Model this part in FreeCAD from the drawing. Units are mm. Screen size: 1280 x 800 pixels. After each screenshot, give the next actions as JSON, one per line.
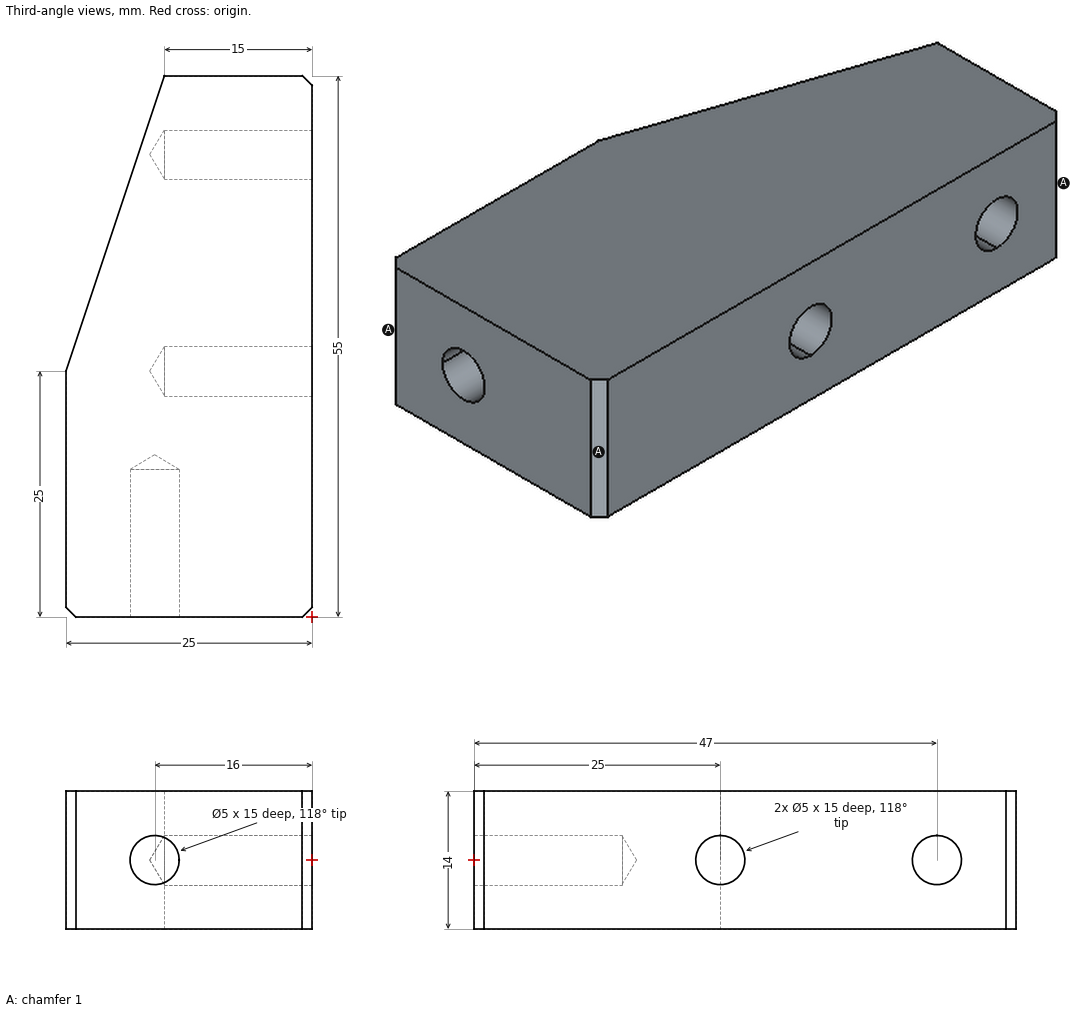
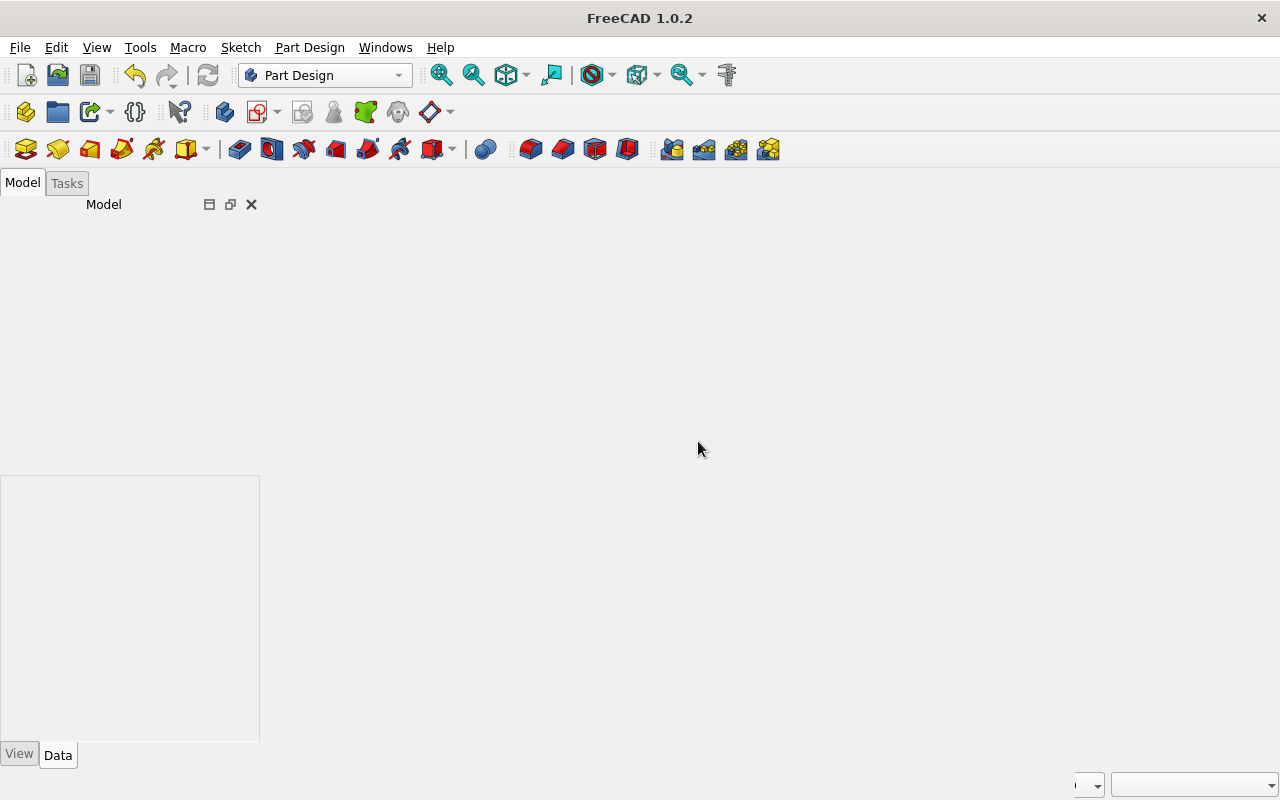
{"action": "key", "text": "ctrl+n"}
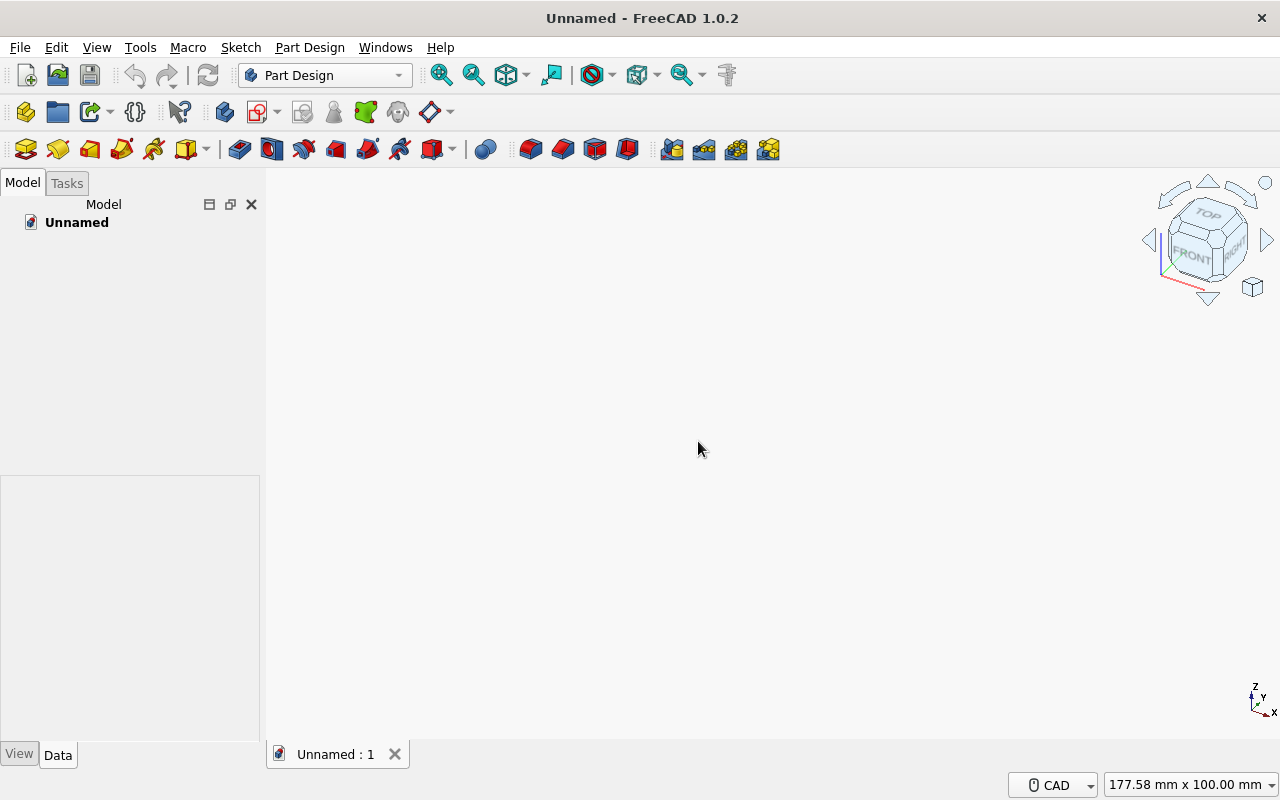
{"action": "left_click", "coordinate": [258, 112]}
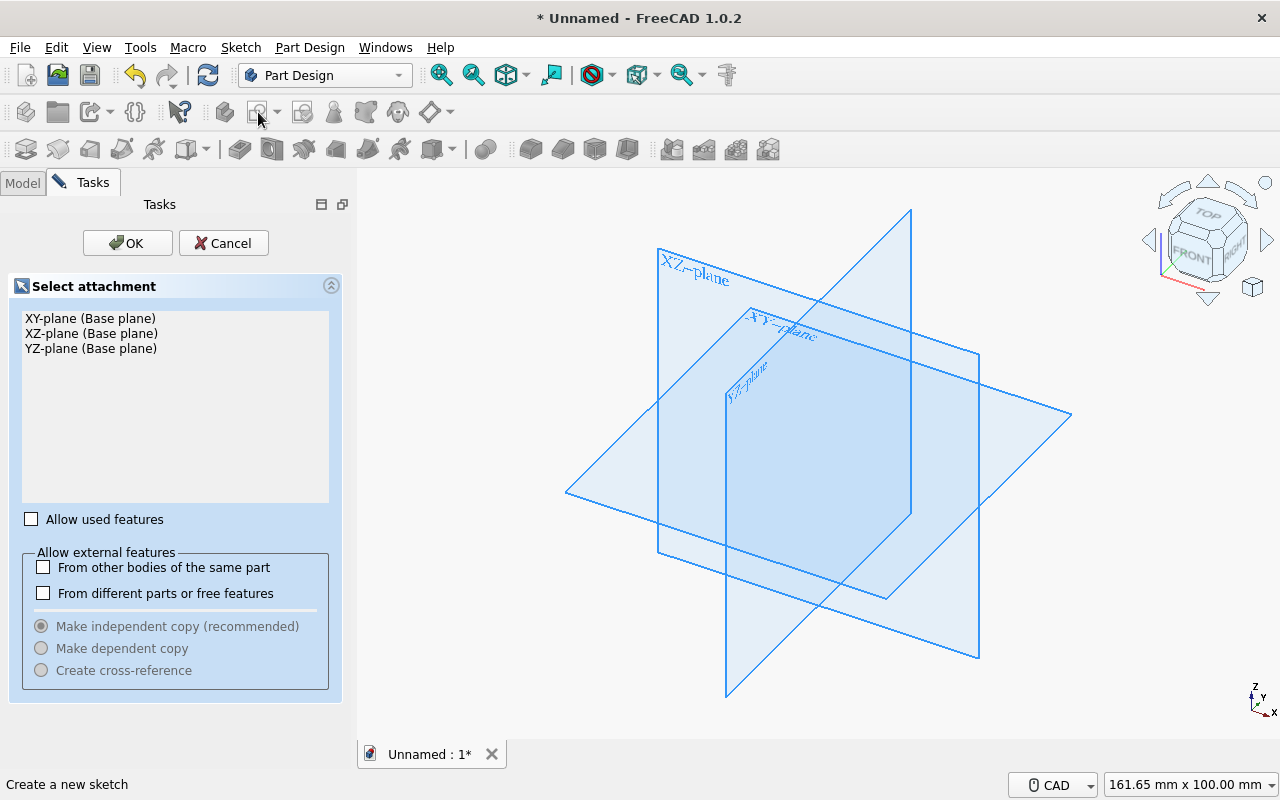
{"action": "left_click", "coordinate": [82, 318]}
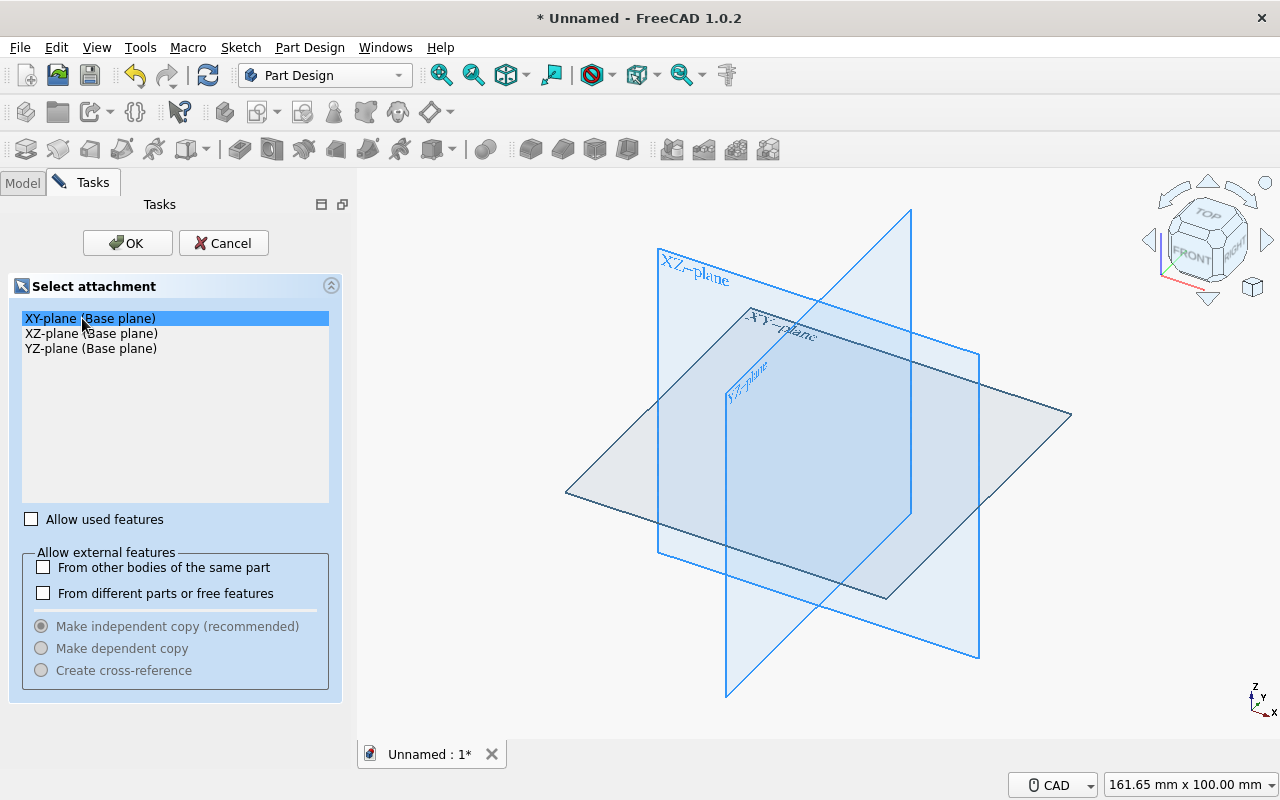
{"action": "left_click", "coordinate": [128, 243]}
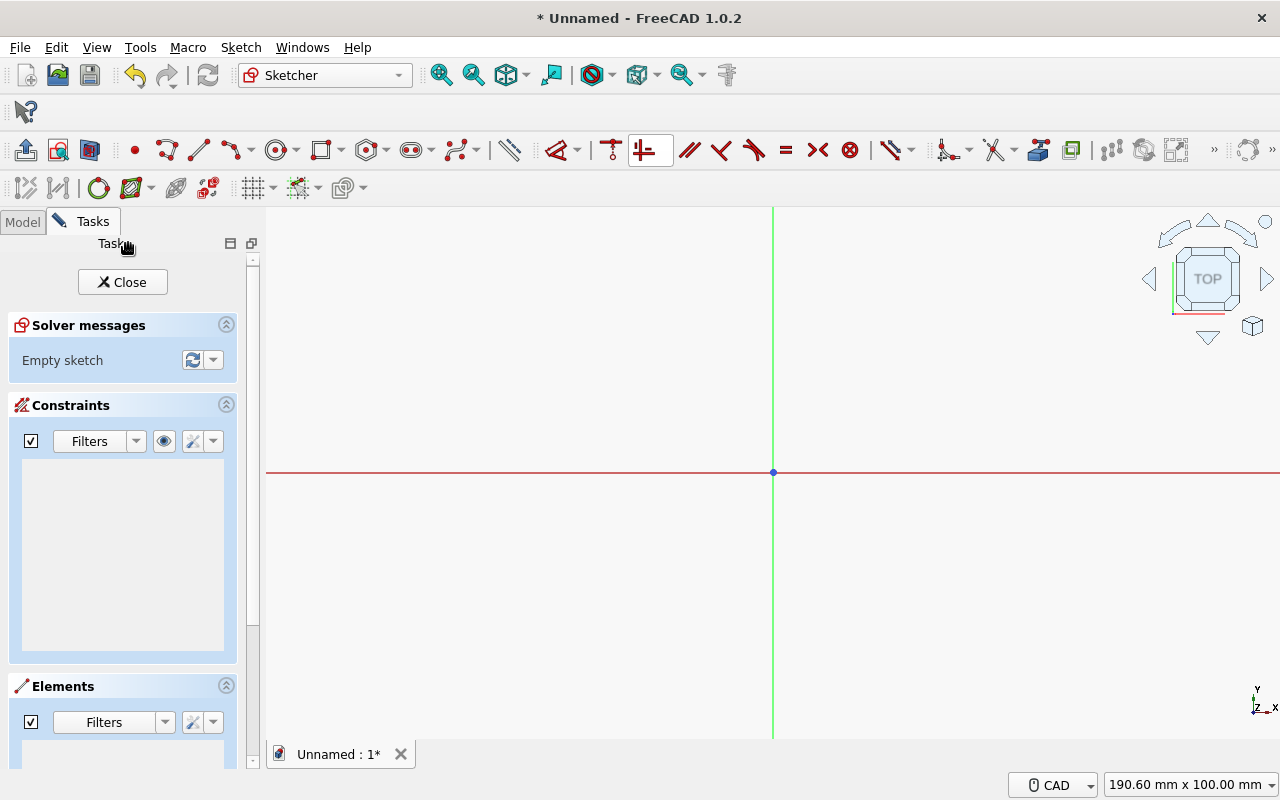
{"action": "scroll", "coordinate": [695, 711], "scroll_direction": "down", "scroll_amount": 1}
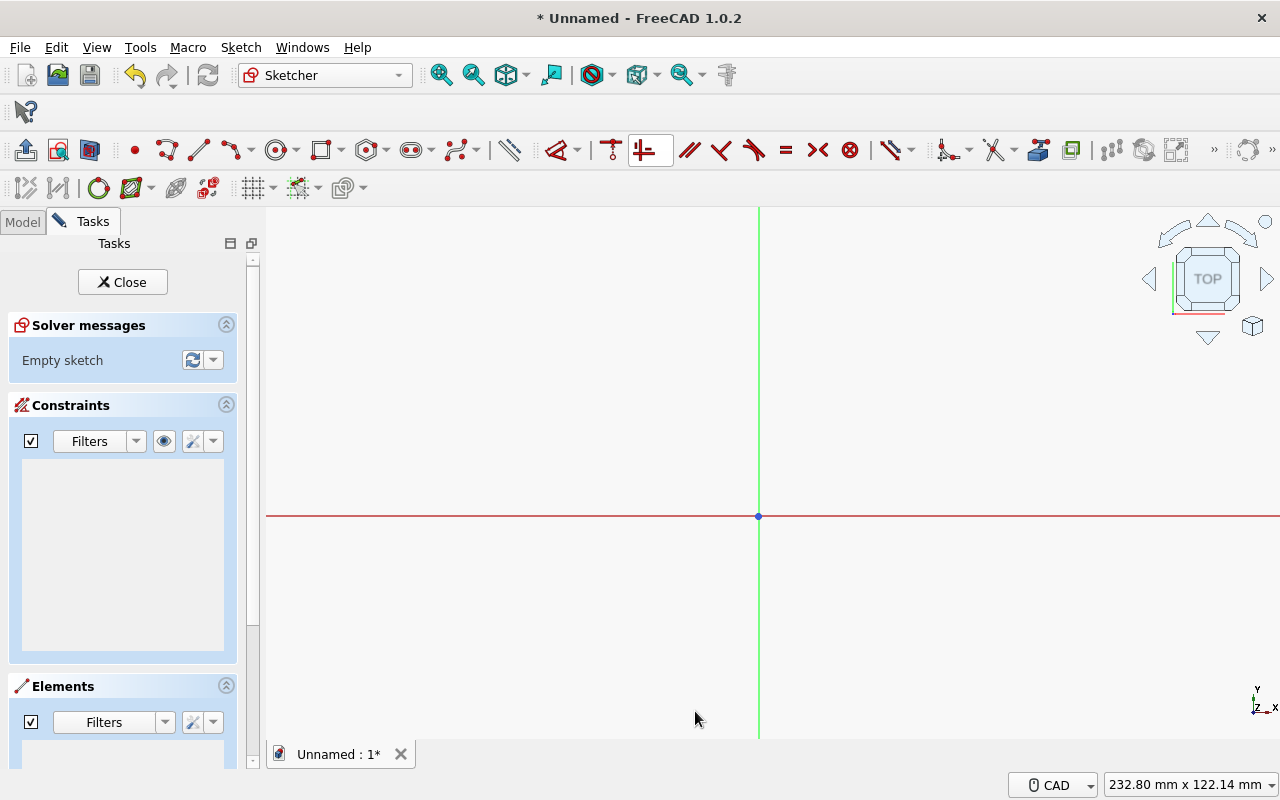
{"action": "scroll", "coordinate": [704, 241], "scroll_direction": "up", "scroll_amount": 2}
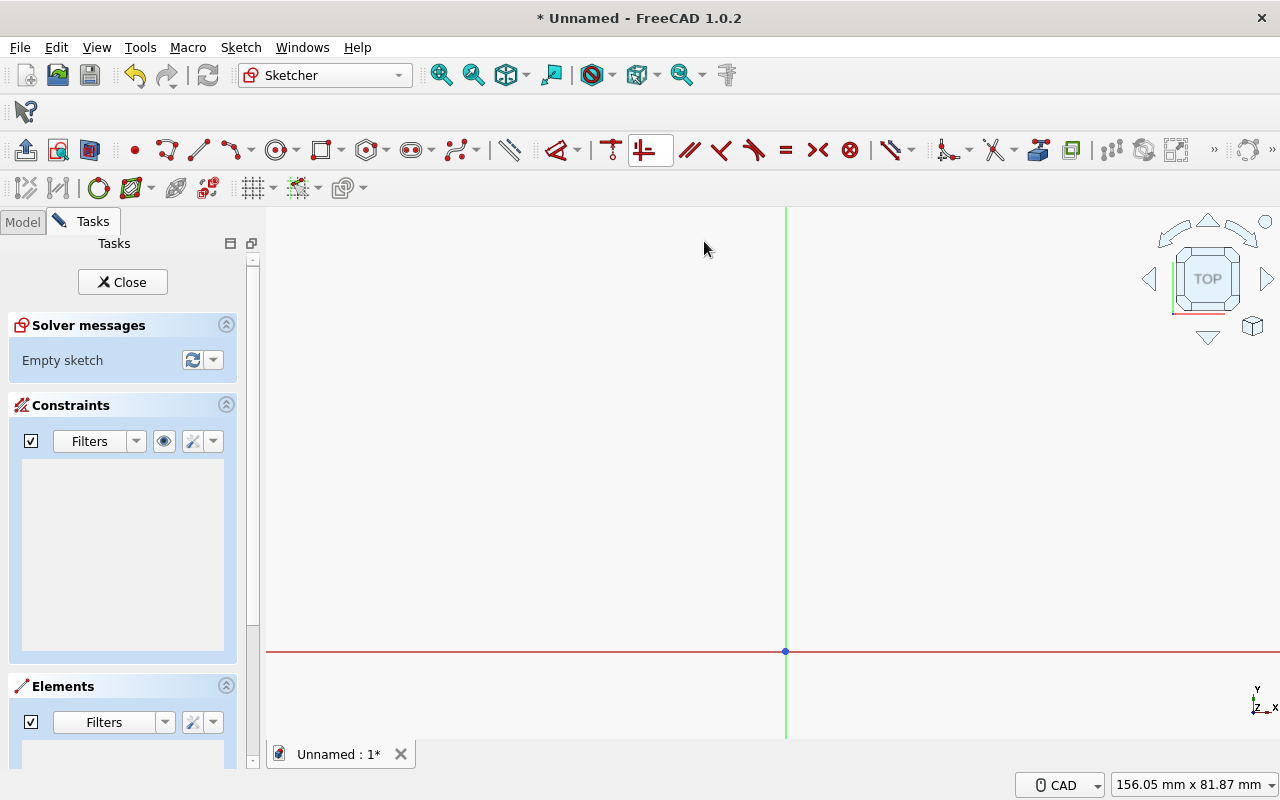
{"action": "key", "text": "g m"}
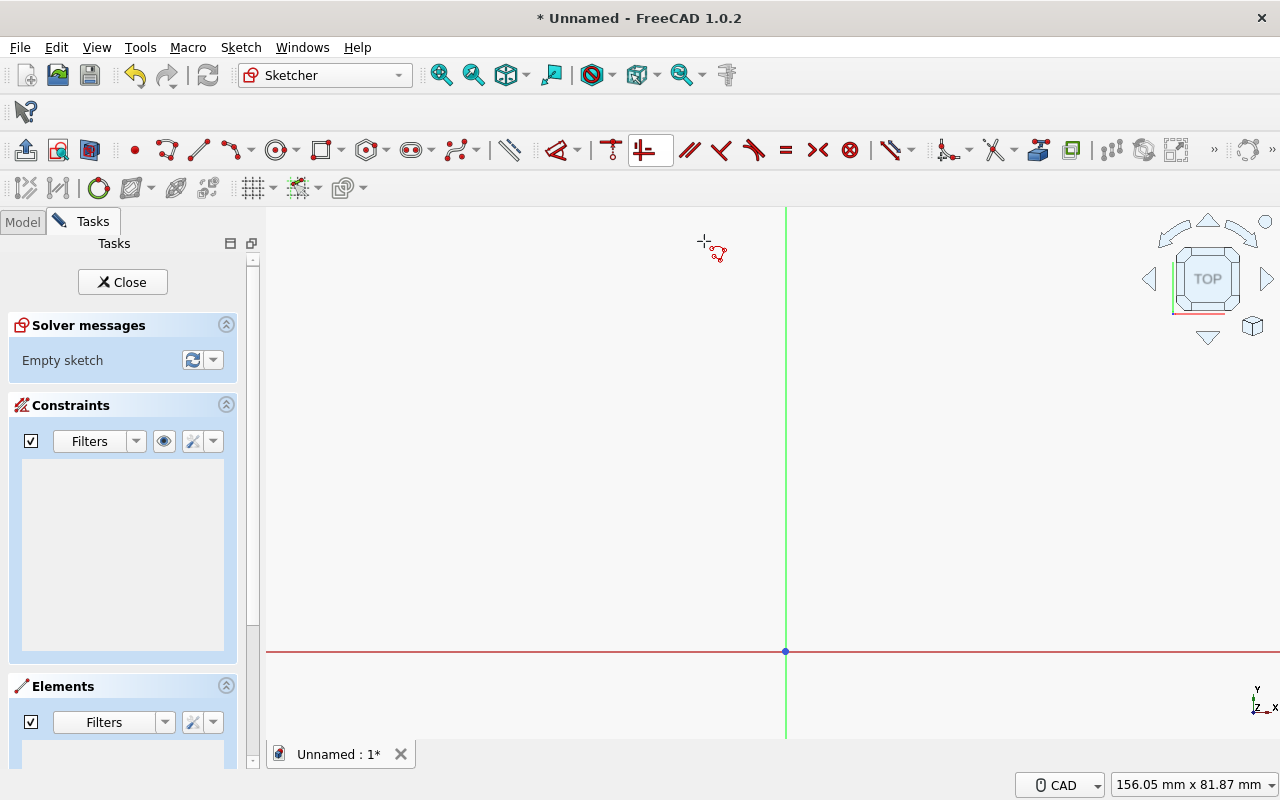
{"action": "left_click", "coordinate": [786, 652]}
{"action": "left_click", "coordinate": [777, 294]}
{"action": "left_click", "coordinate": [688, 294]}
{"action": "left_click", "coordinate": [623, 489]}
{"action": "left_click", "coordinate": [623, 643]}
{"action": "left_click", "coordinate": [786, 652]}
{"action": "key", "text": "Escape"}
{"action": "key", "text": "Escape"}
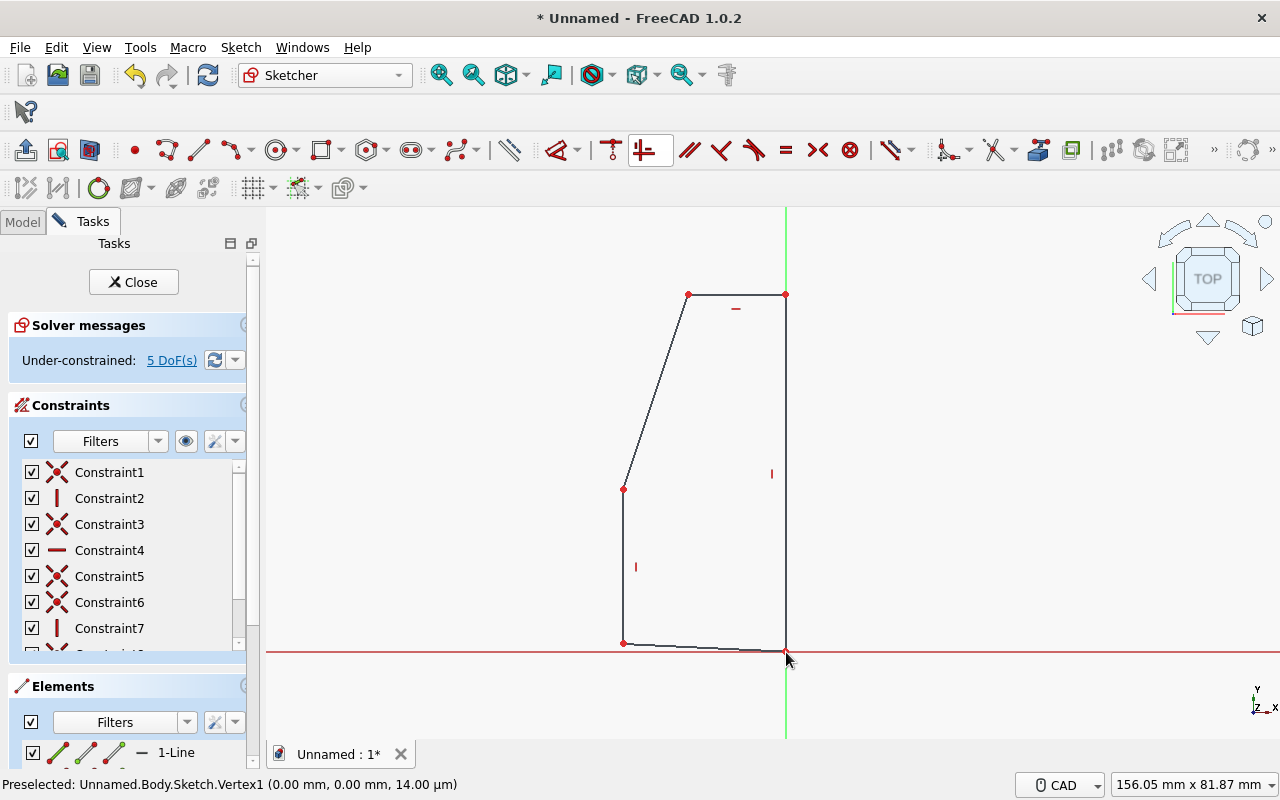
{"action": "left_click", "coordinate": [737, 649]}